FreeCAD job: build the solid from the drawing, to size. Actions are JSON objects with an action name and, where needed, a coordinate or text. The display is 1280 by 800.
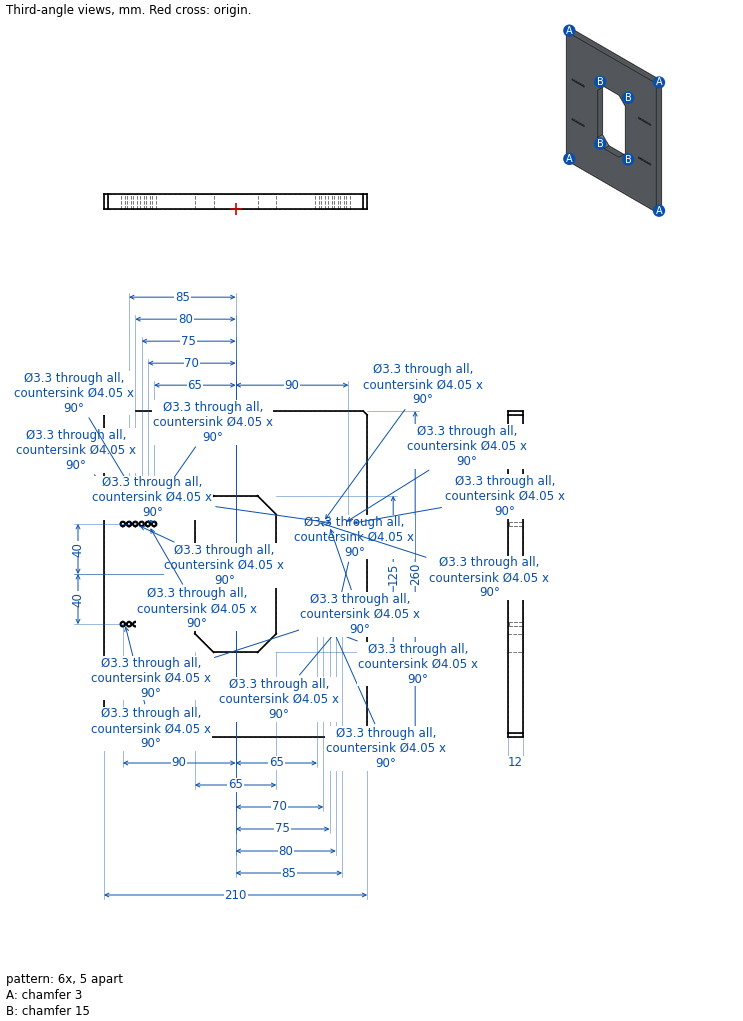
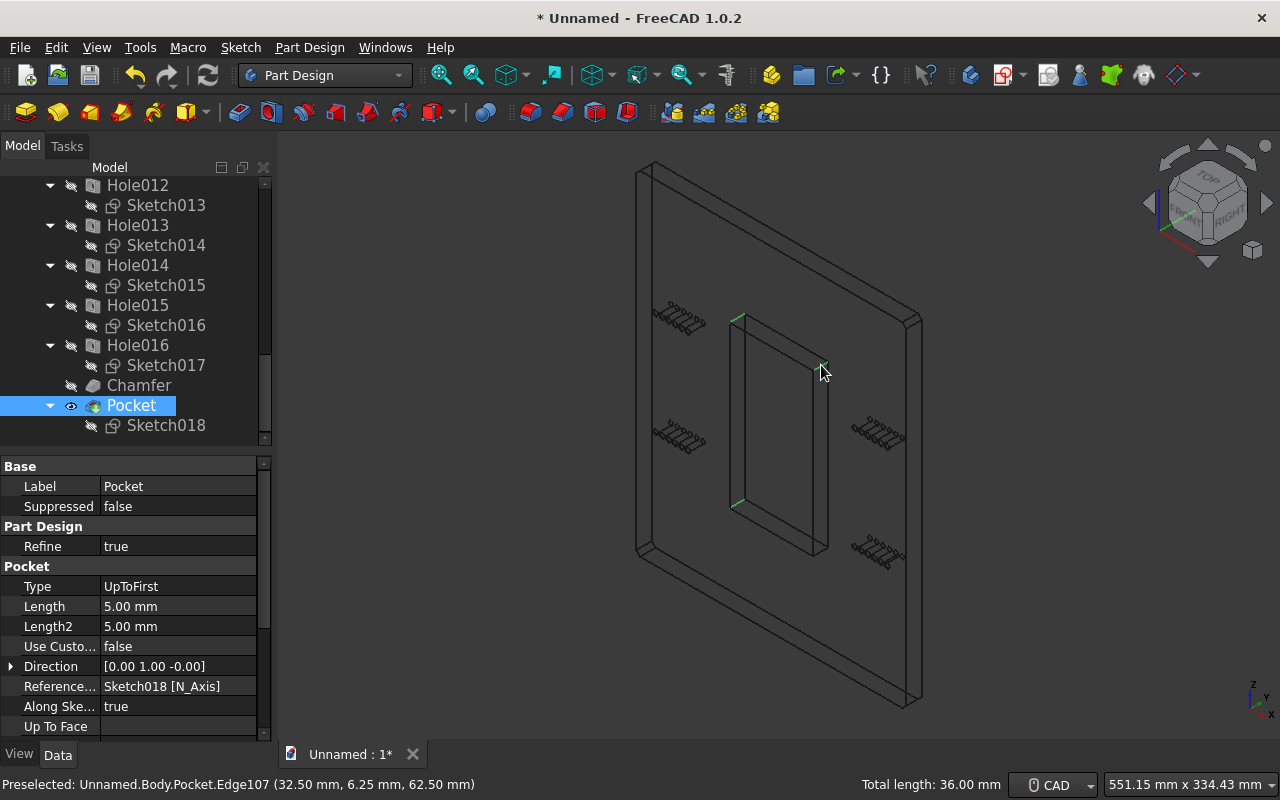
{"action": "left_click", "coordinate": [821, 551], "text": "ctrl"}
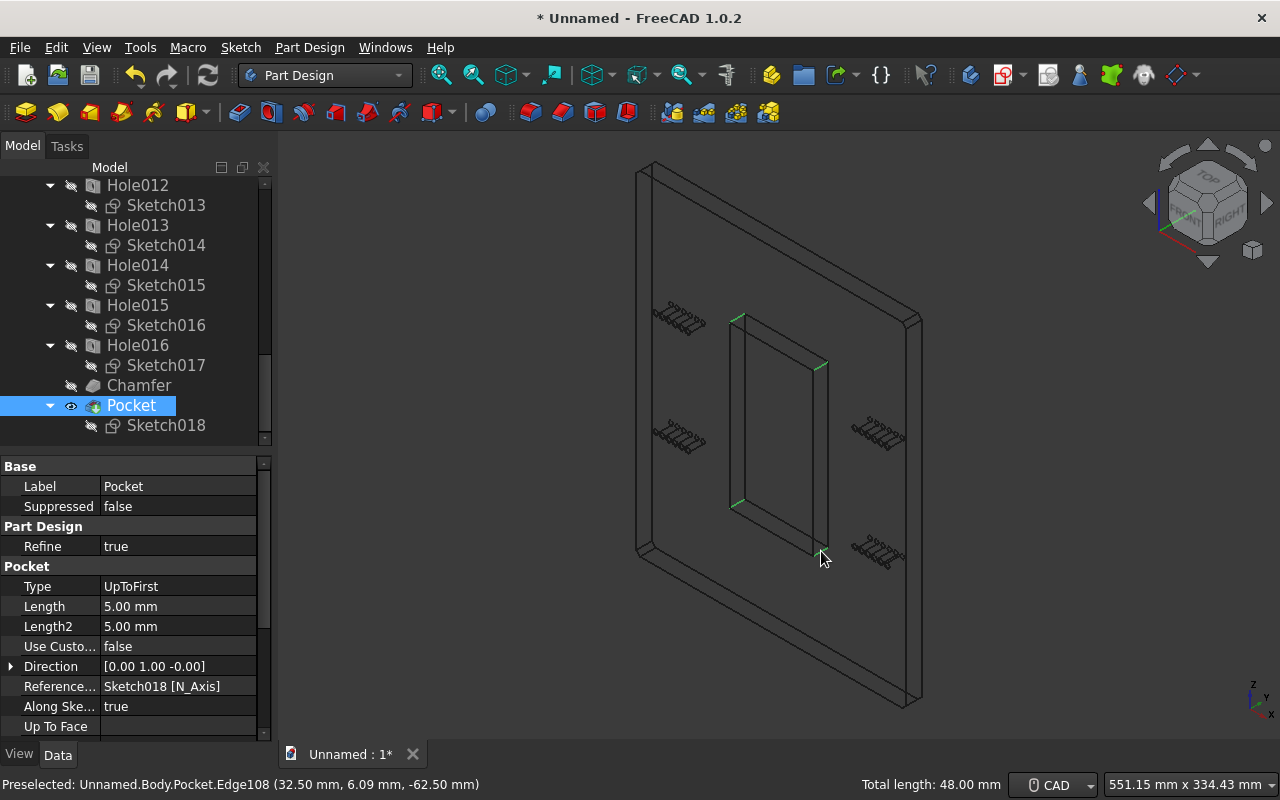
{"action": "key", "text": "v 1"}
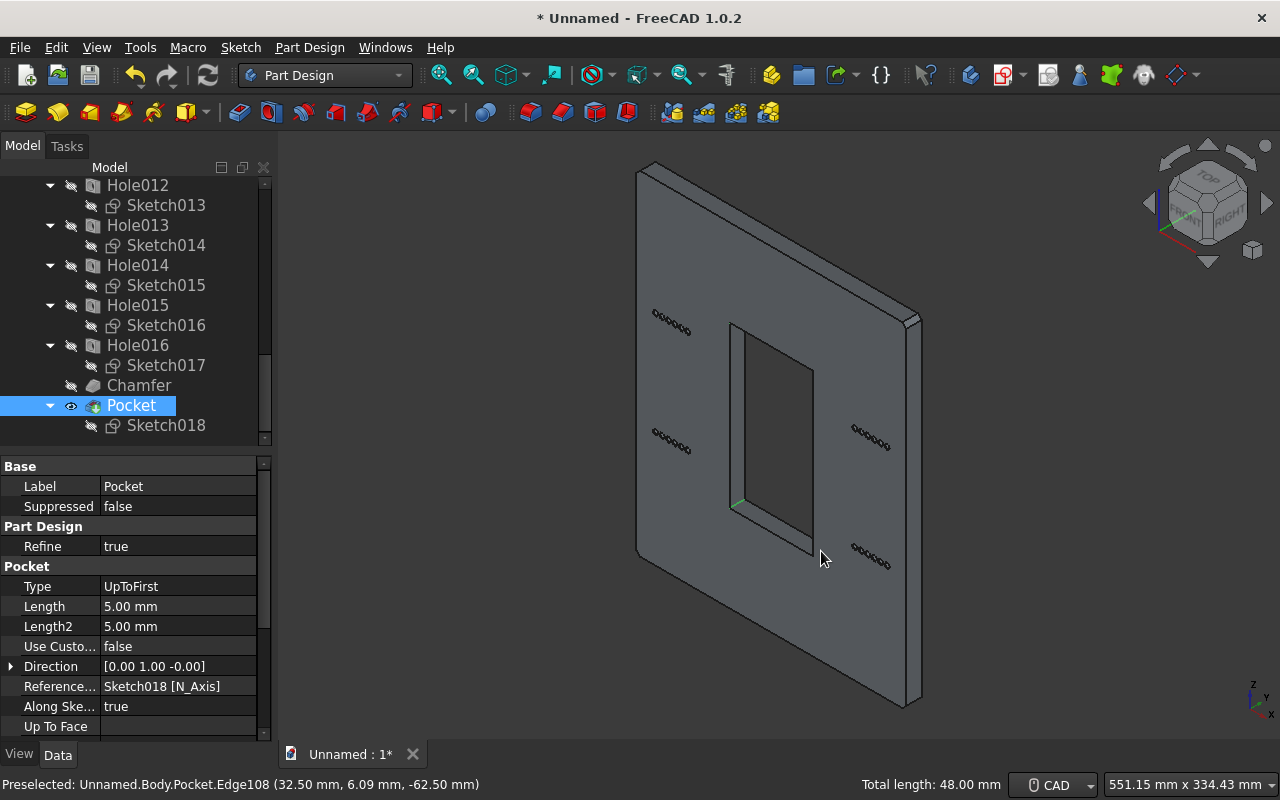
{"action": "left_click", "coordinate": [564, 112]}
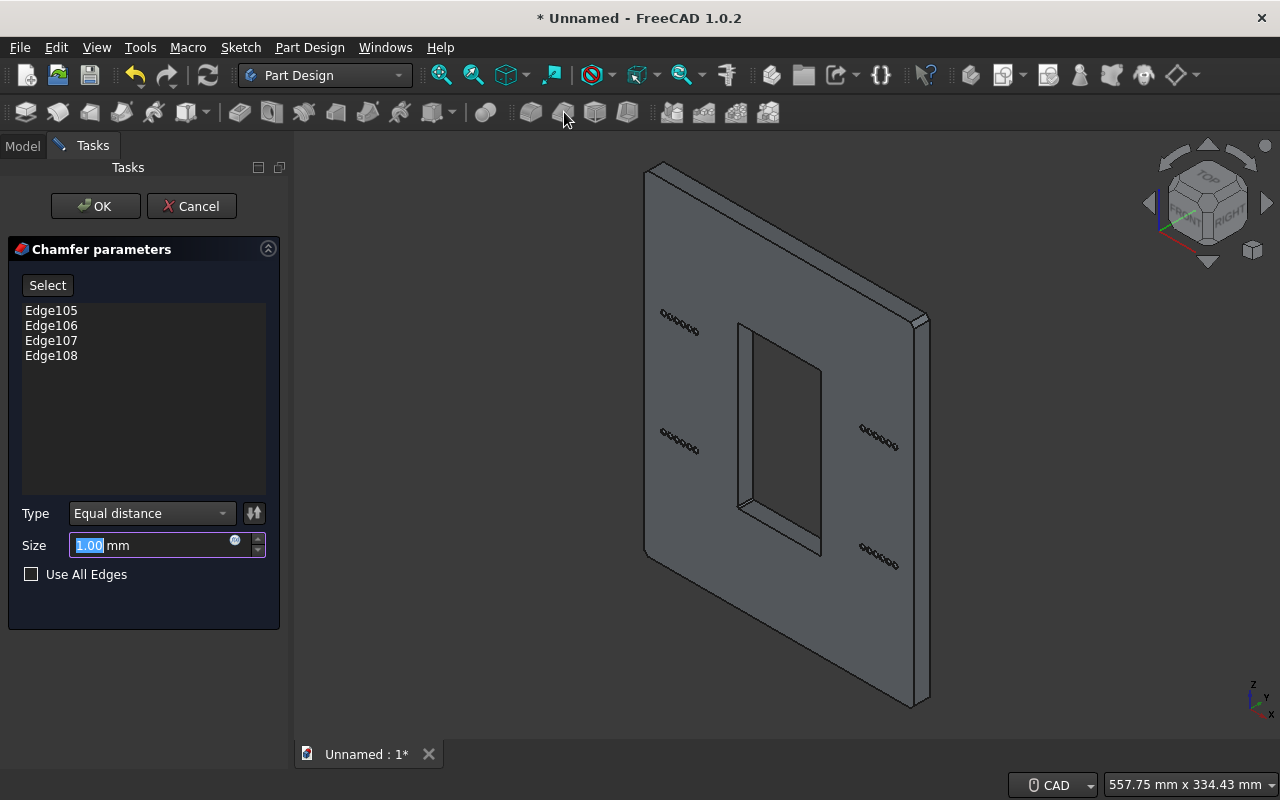
{"action": "type", "text": "15"}
{"action": "key", "text": "Tab"}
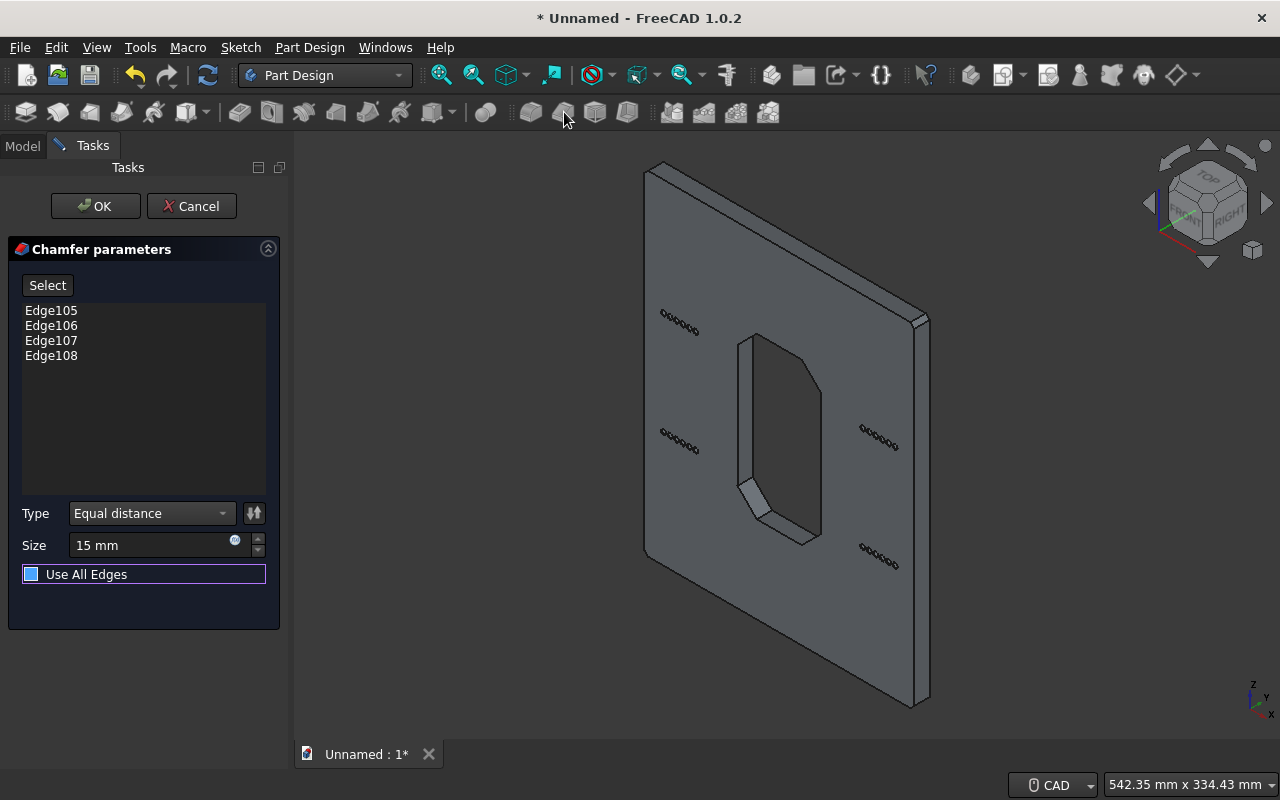
{"action": "left_click", "coordinate": [96, 206]}